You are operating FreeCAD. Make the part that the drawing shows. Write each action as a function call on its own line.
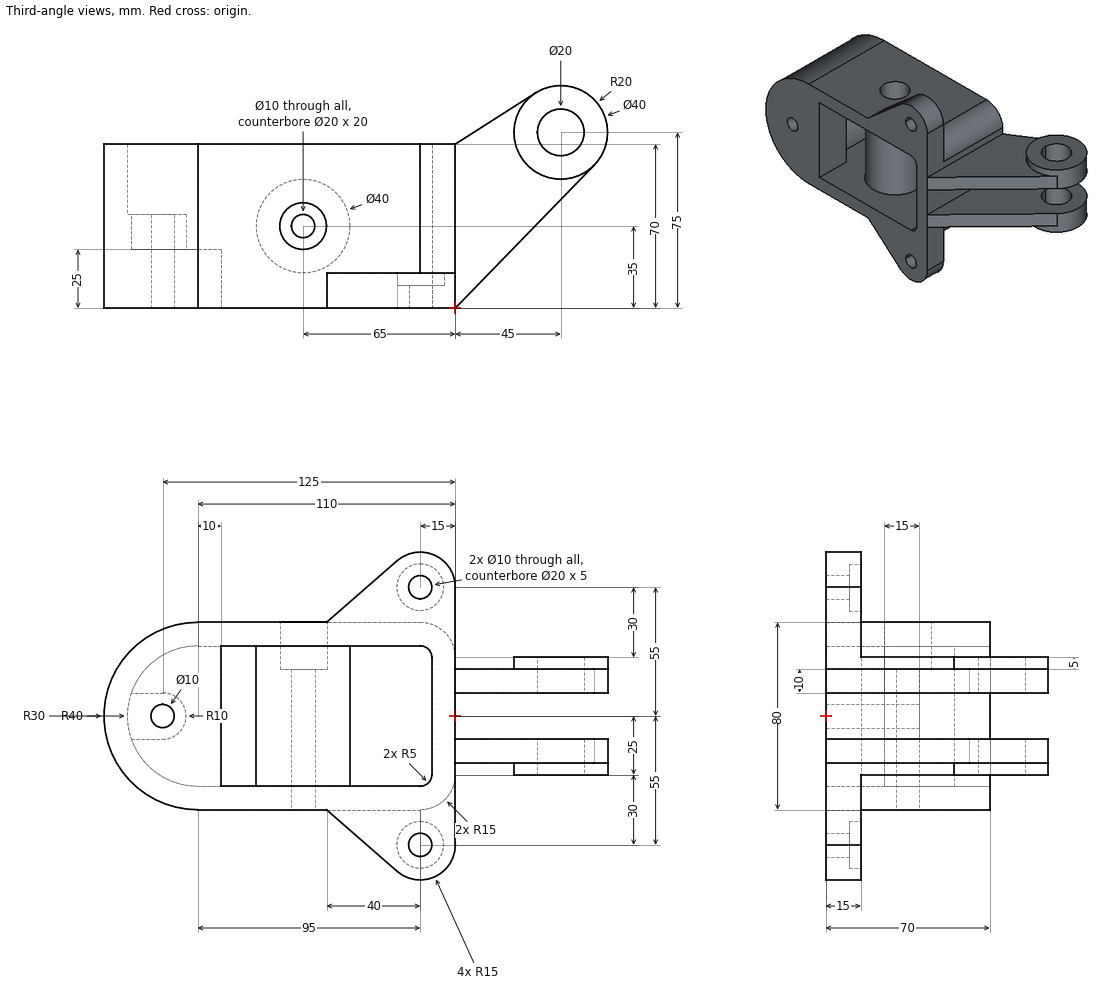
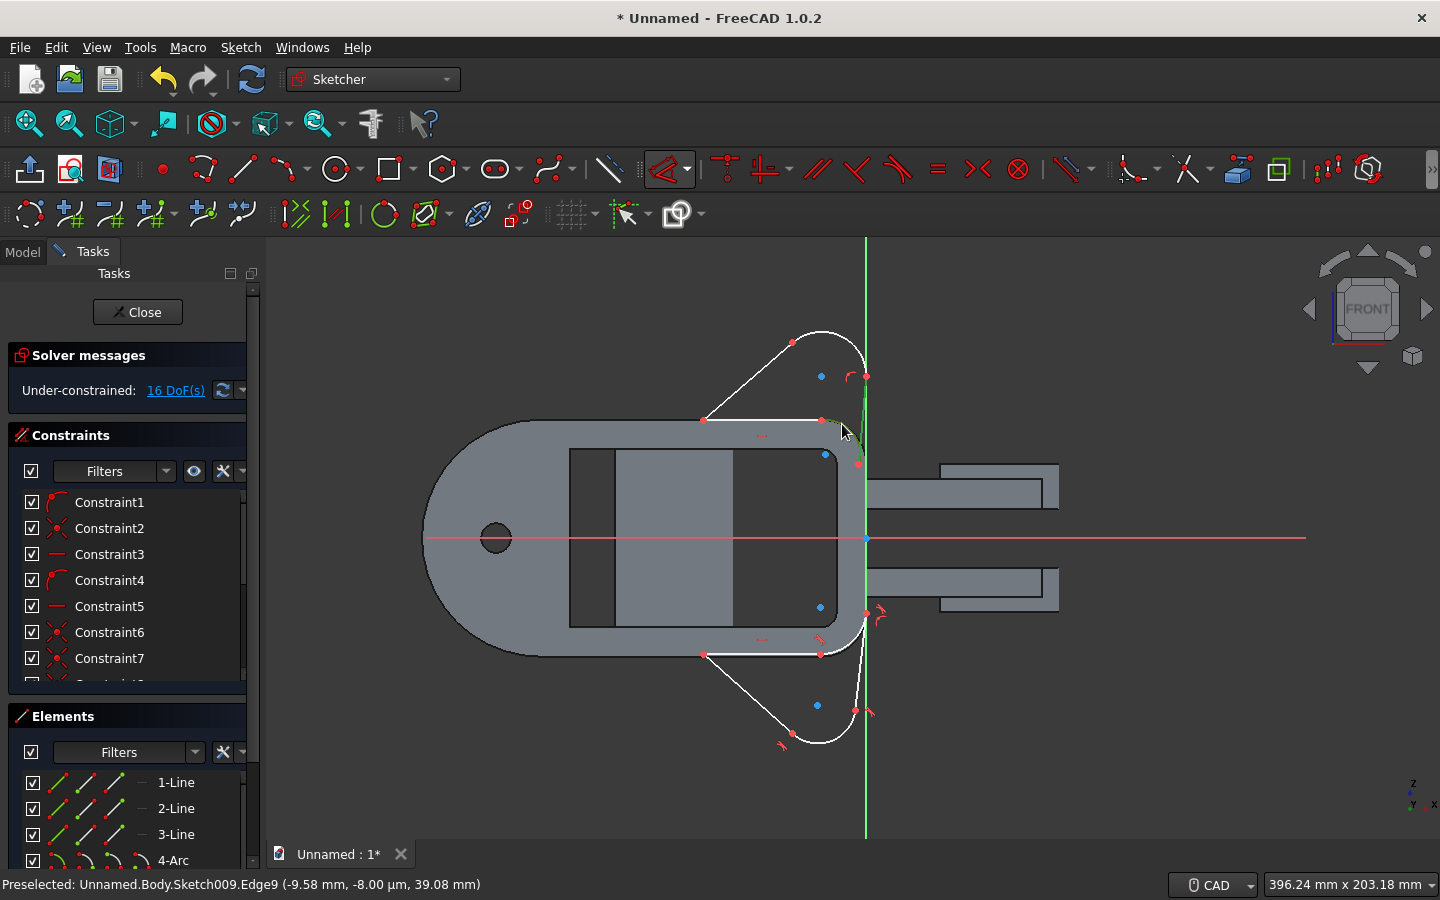
key(t)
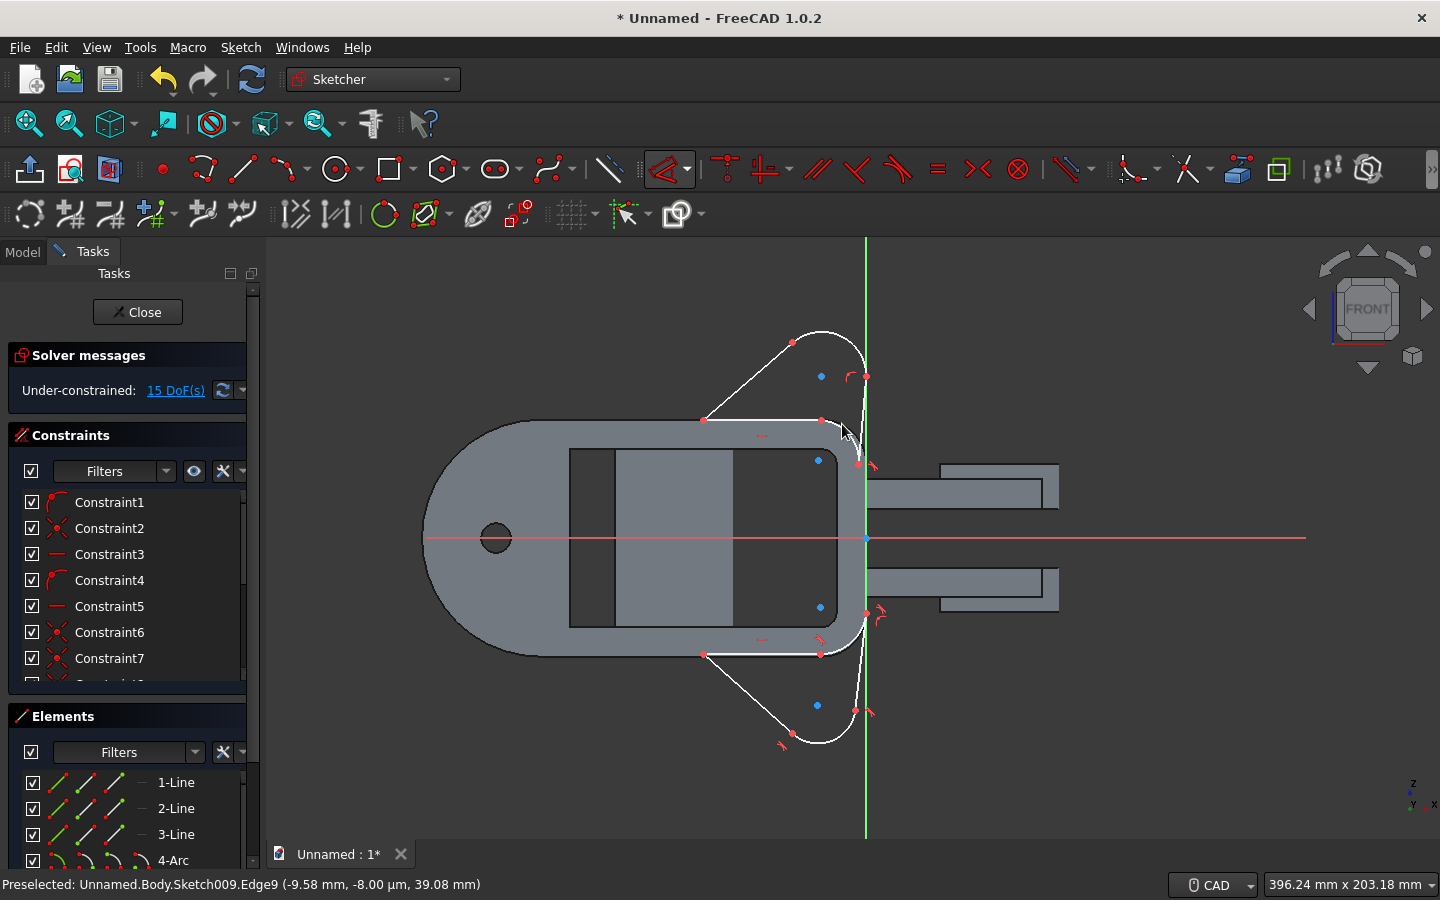
click(864, 403)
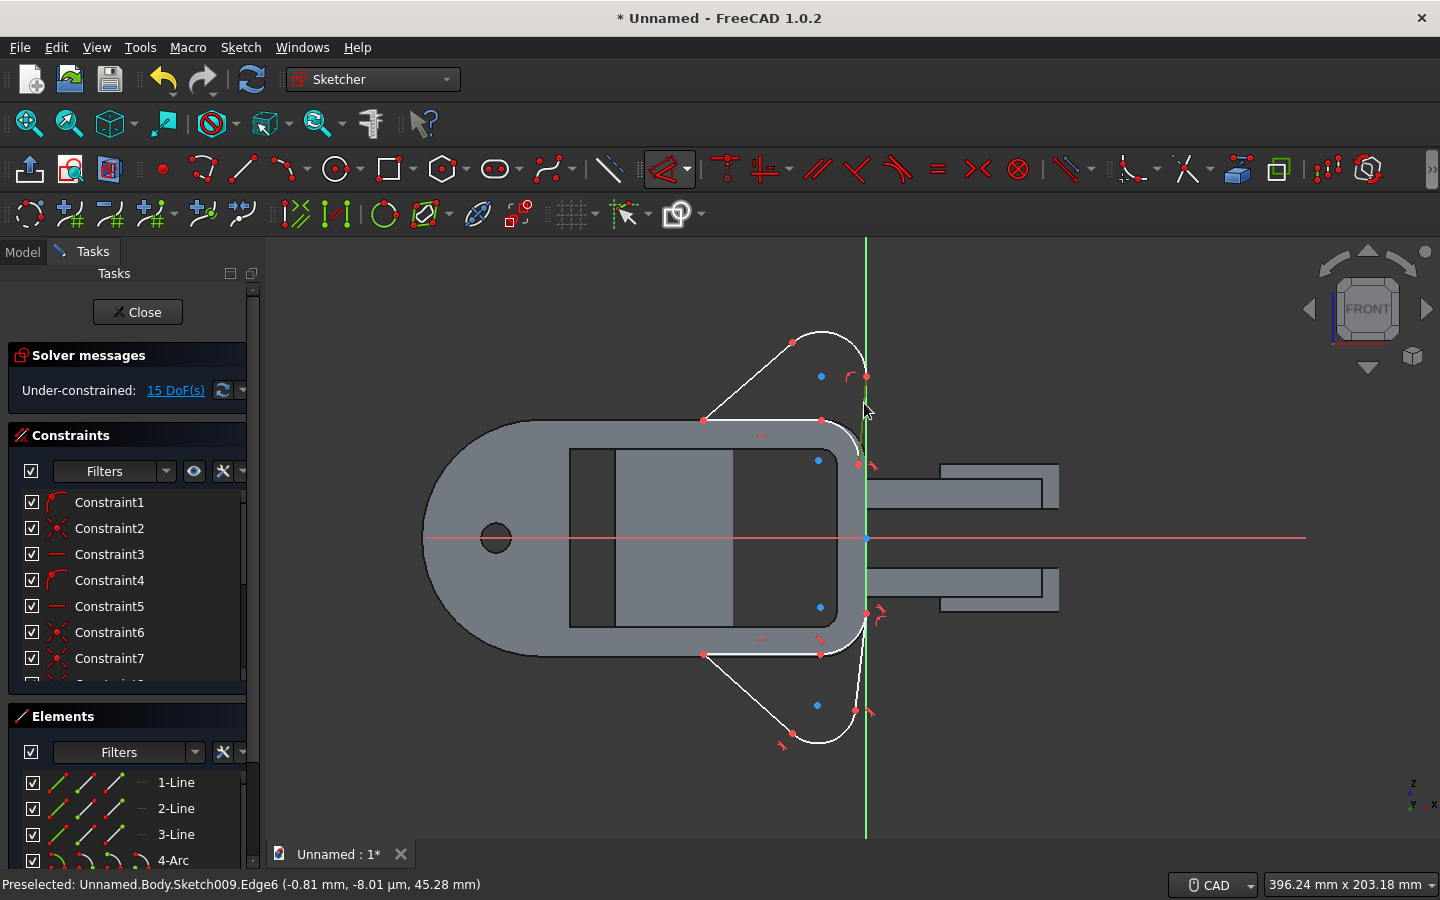
scroll(856, 348, up, 2)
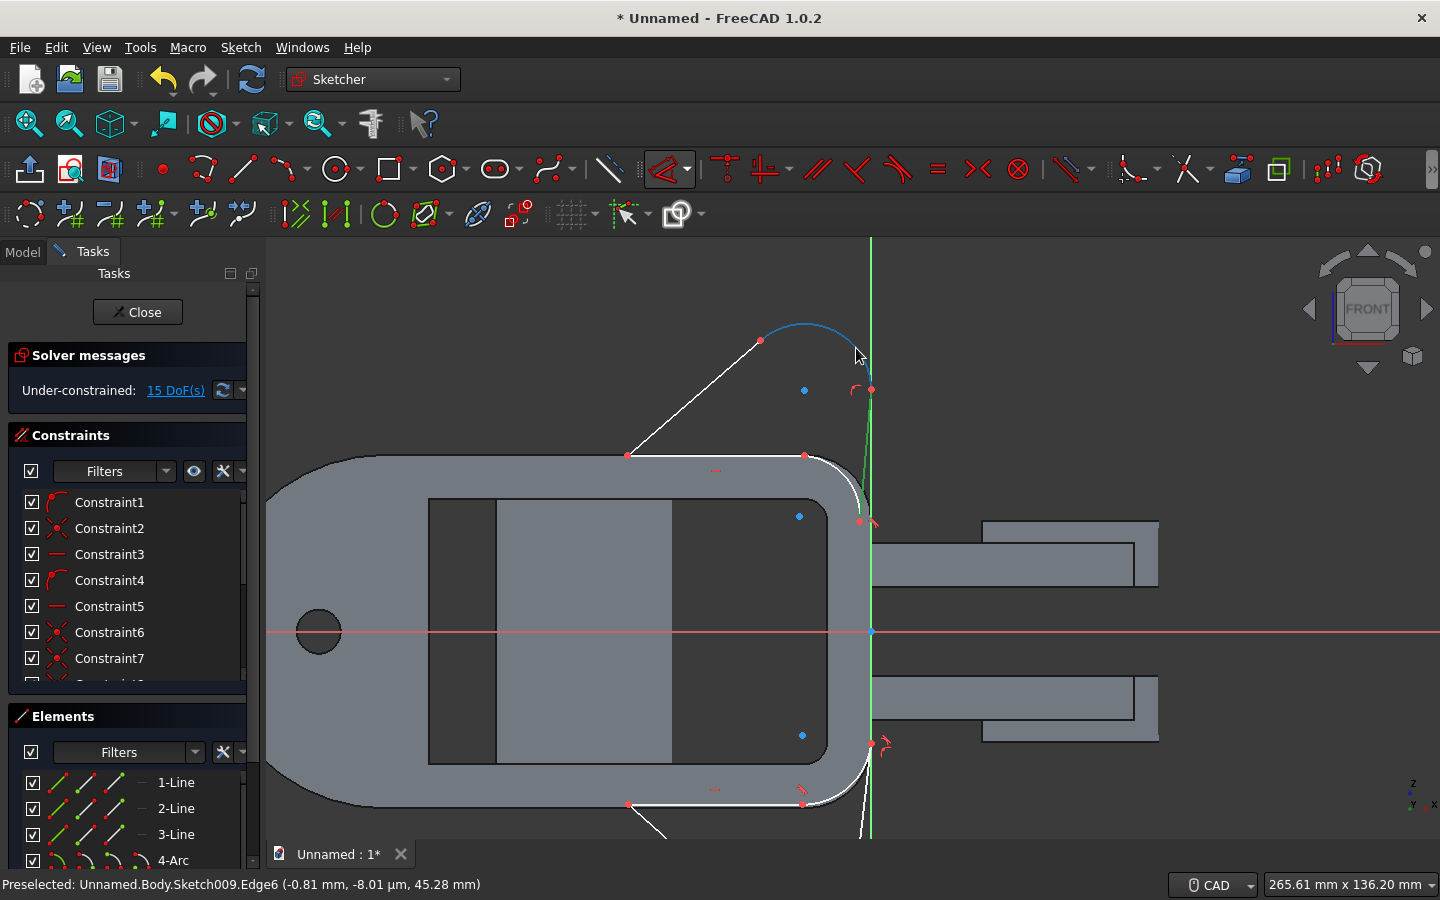
click(856, 348)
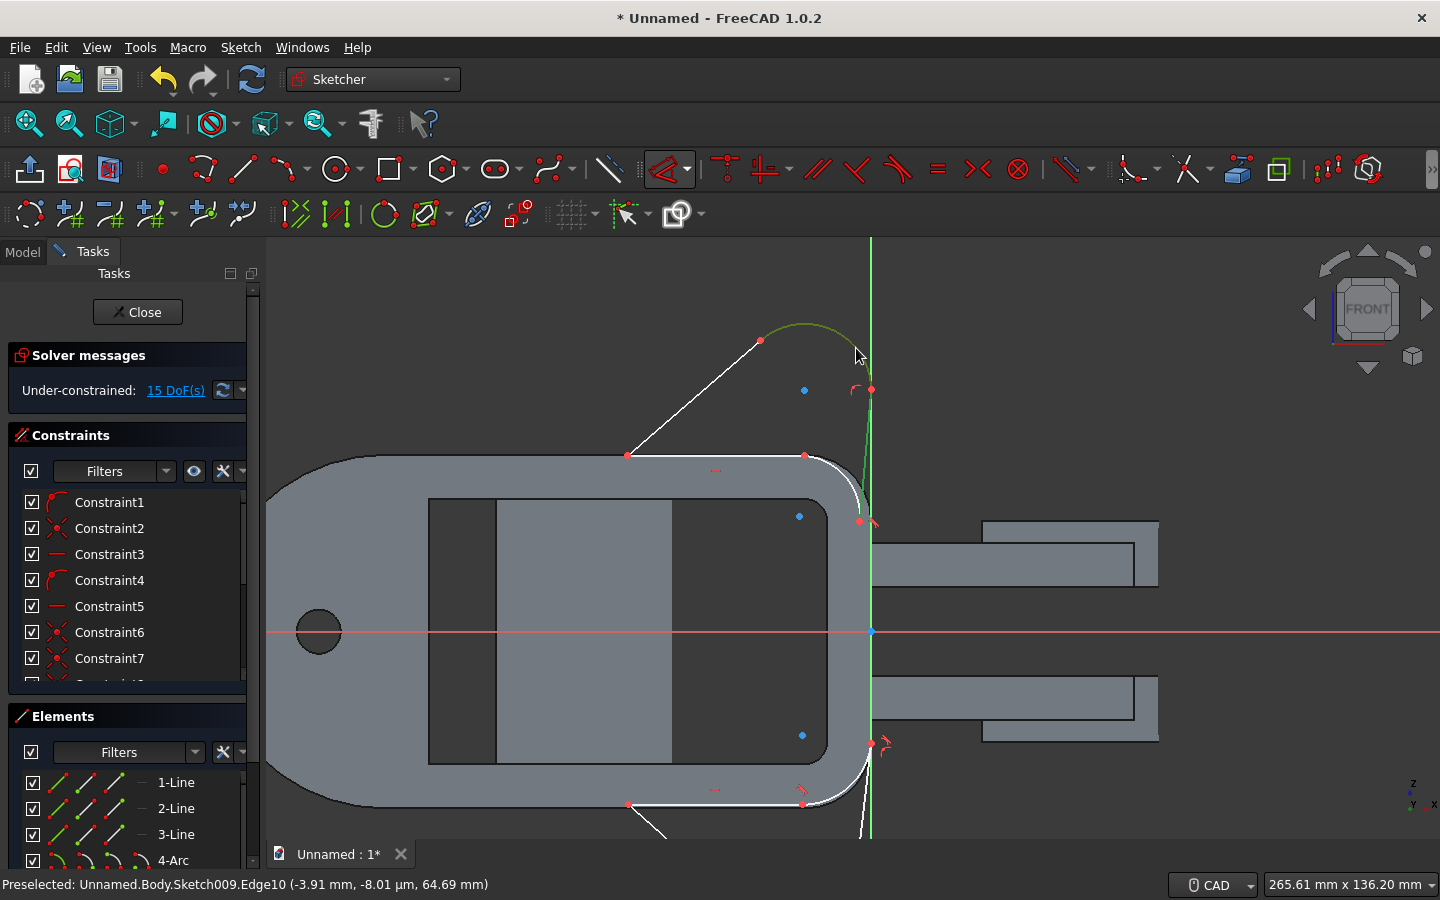
key(t)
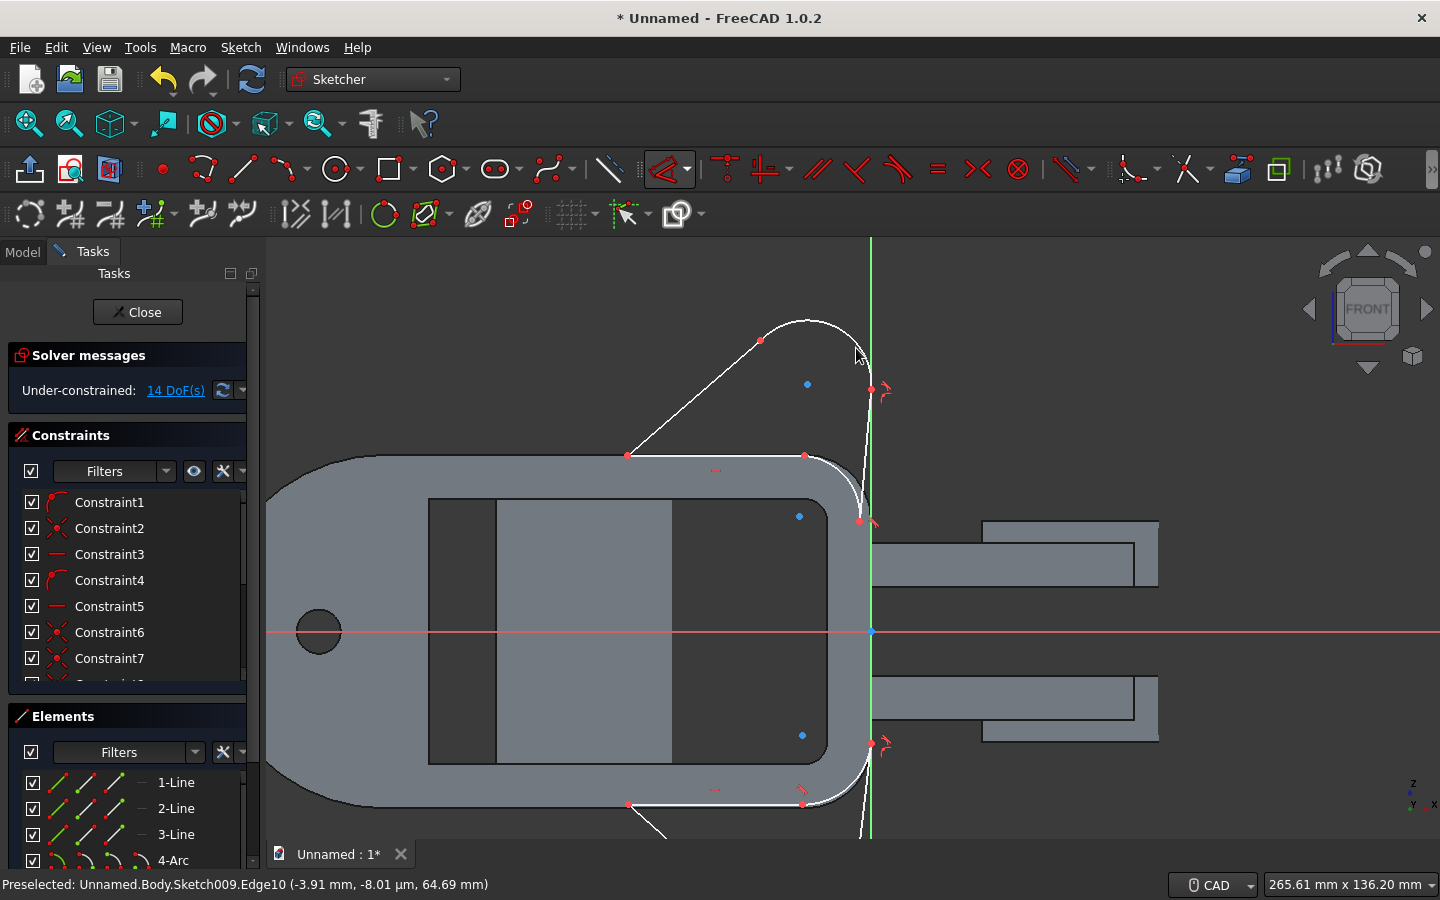
click(752, 456)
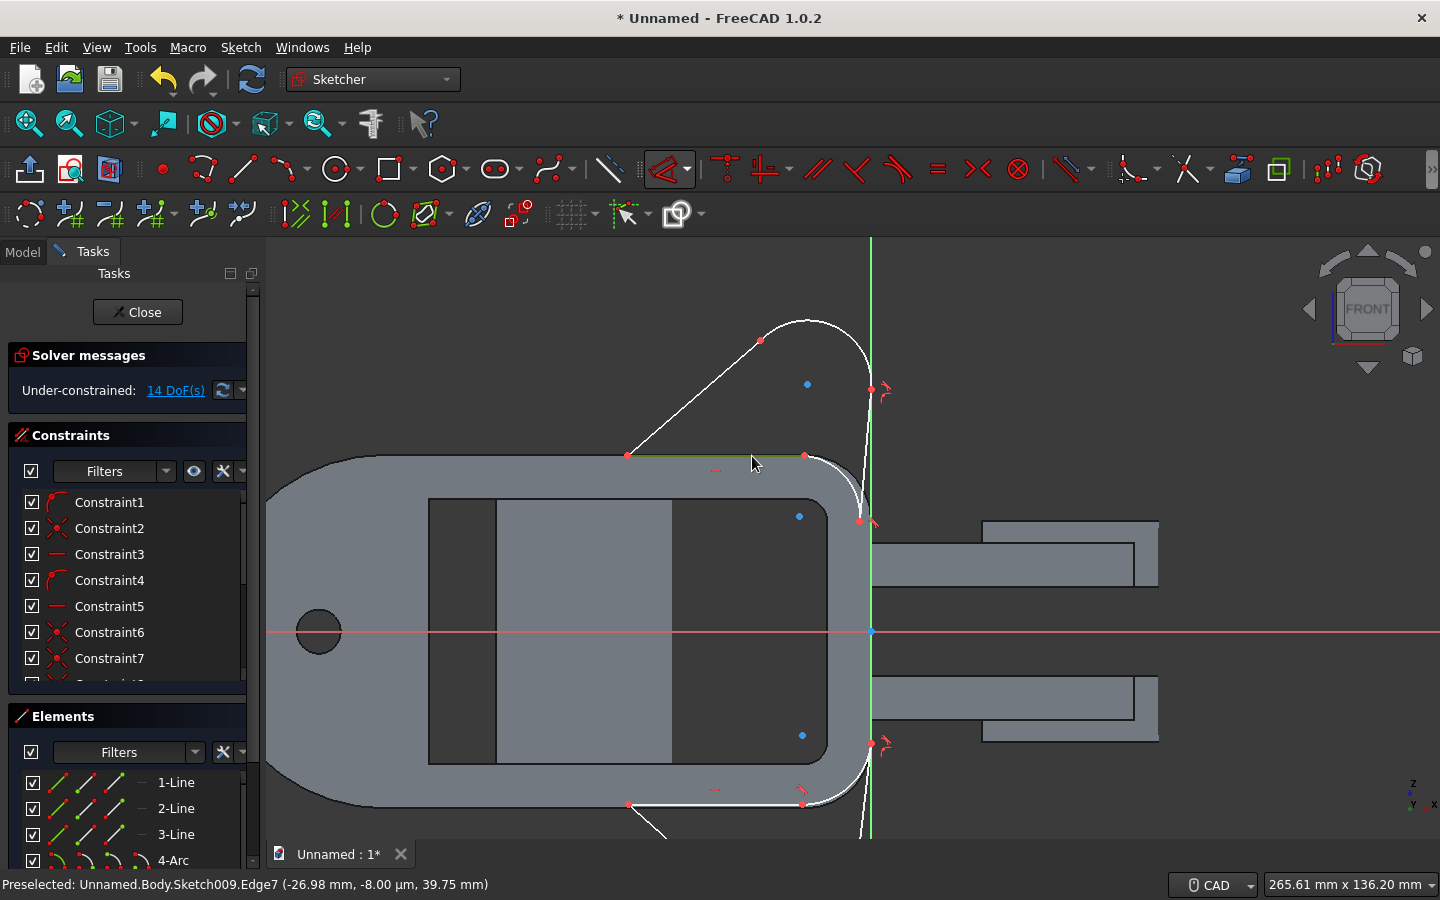
click(832, 465)